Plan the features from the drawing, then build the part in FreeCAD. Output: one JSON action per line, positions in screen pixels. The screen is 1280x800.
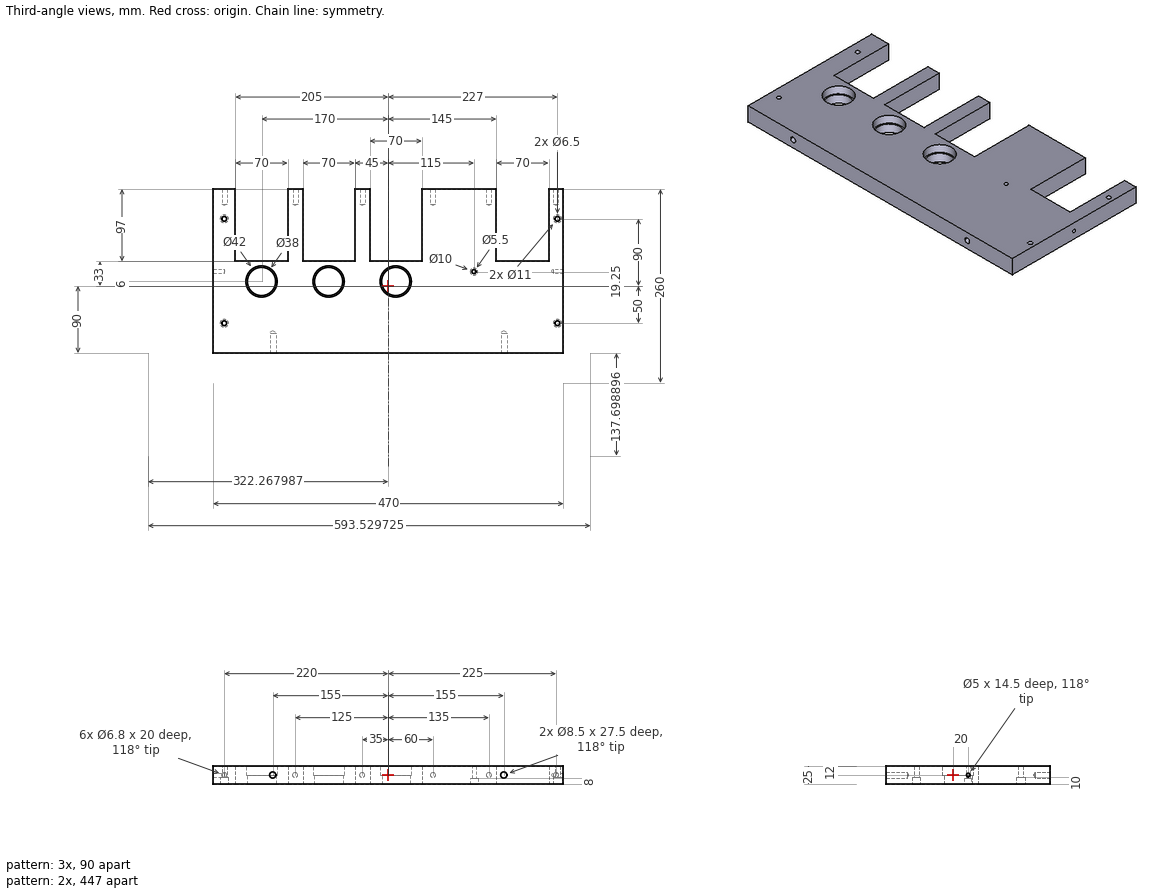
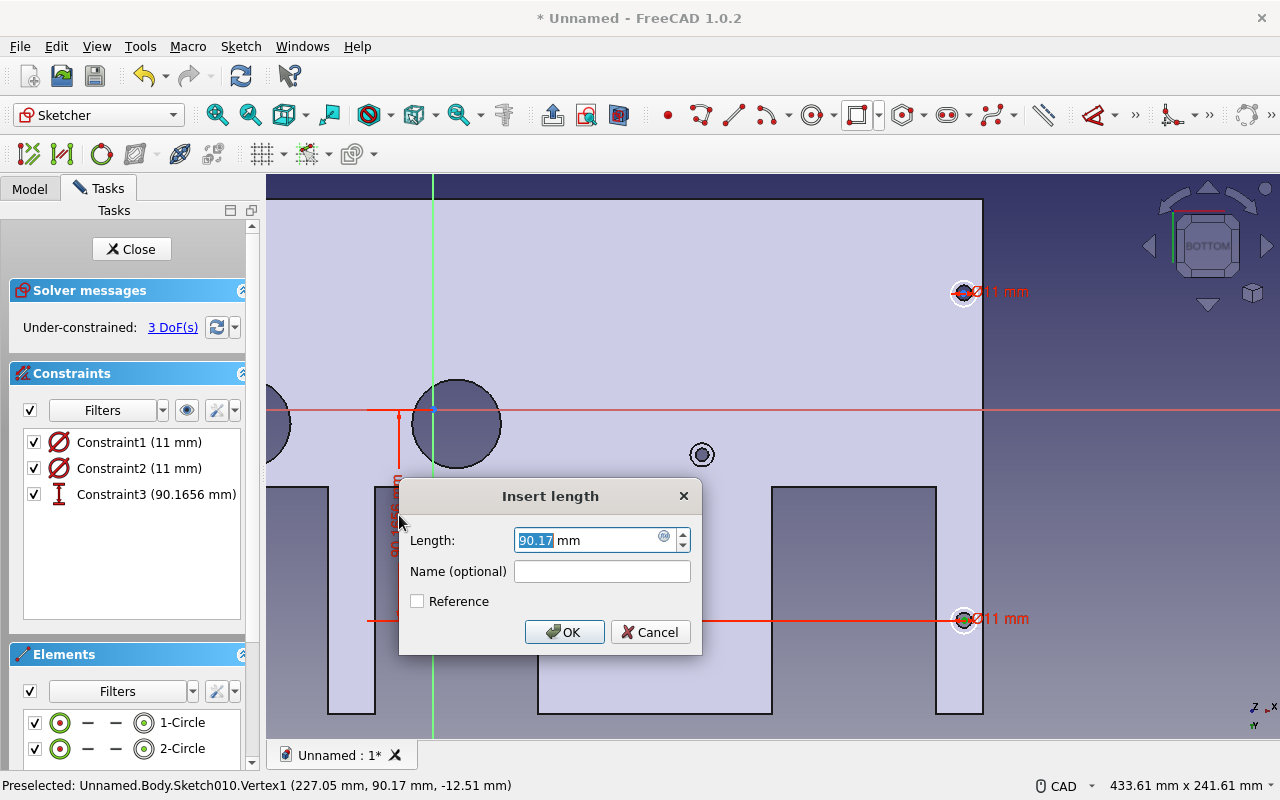
{"action": "type", "text": "90"}
{"action": "key", "text": "Return"}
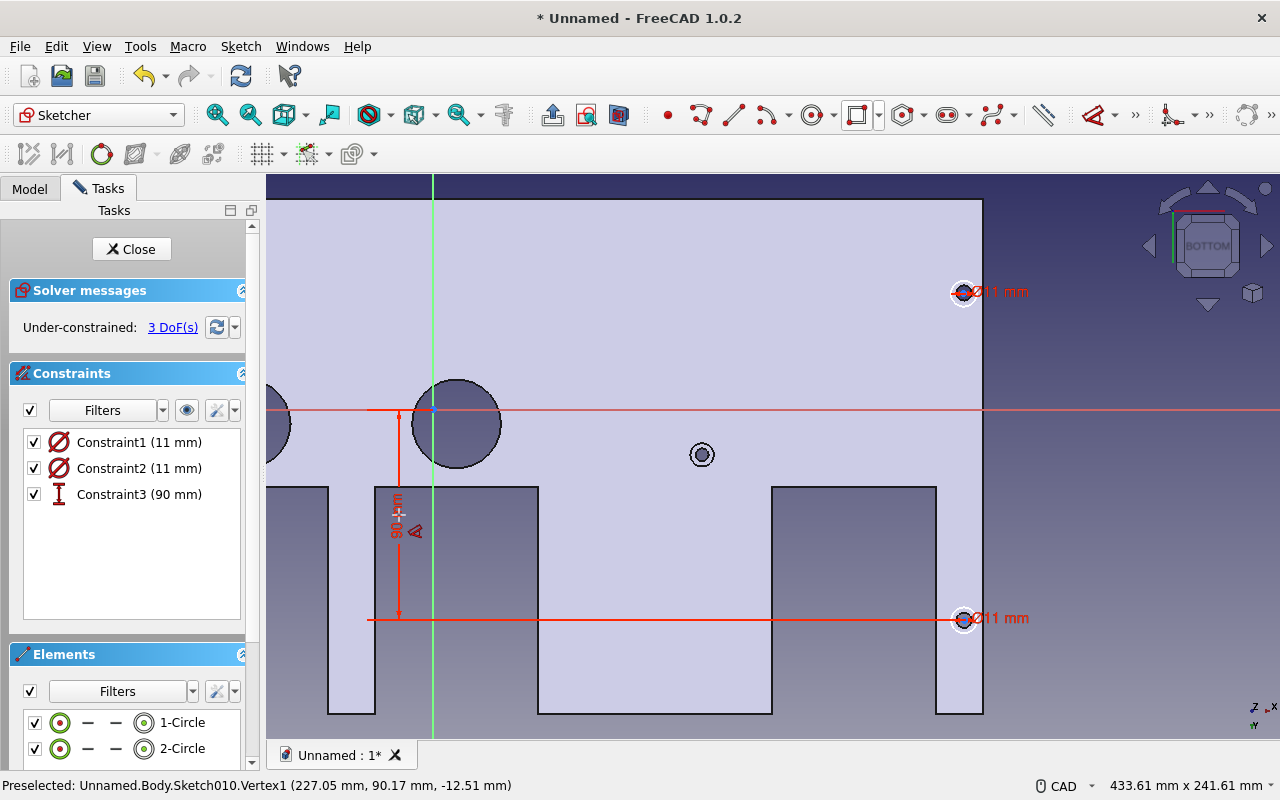
{"action": "left_click", "coordinate": [964, 294]}
{"action": "left_click", "coordinate": [399, 352]}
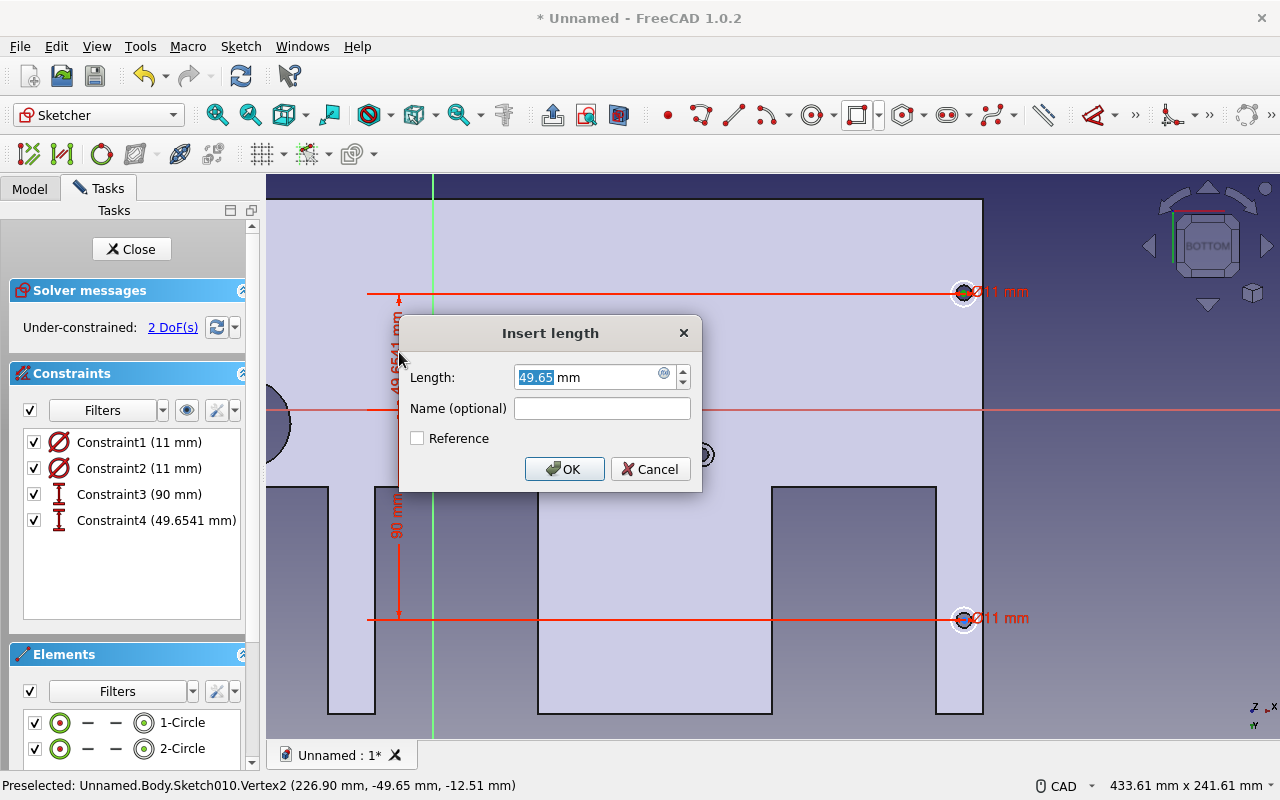
{"action": "type", "text": "50"}
{"action": "key", "text": "Return"}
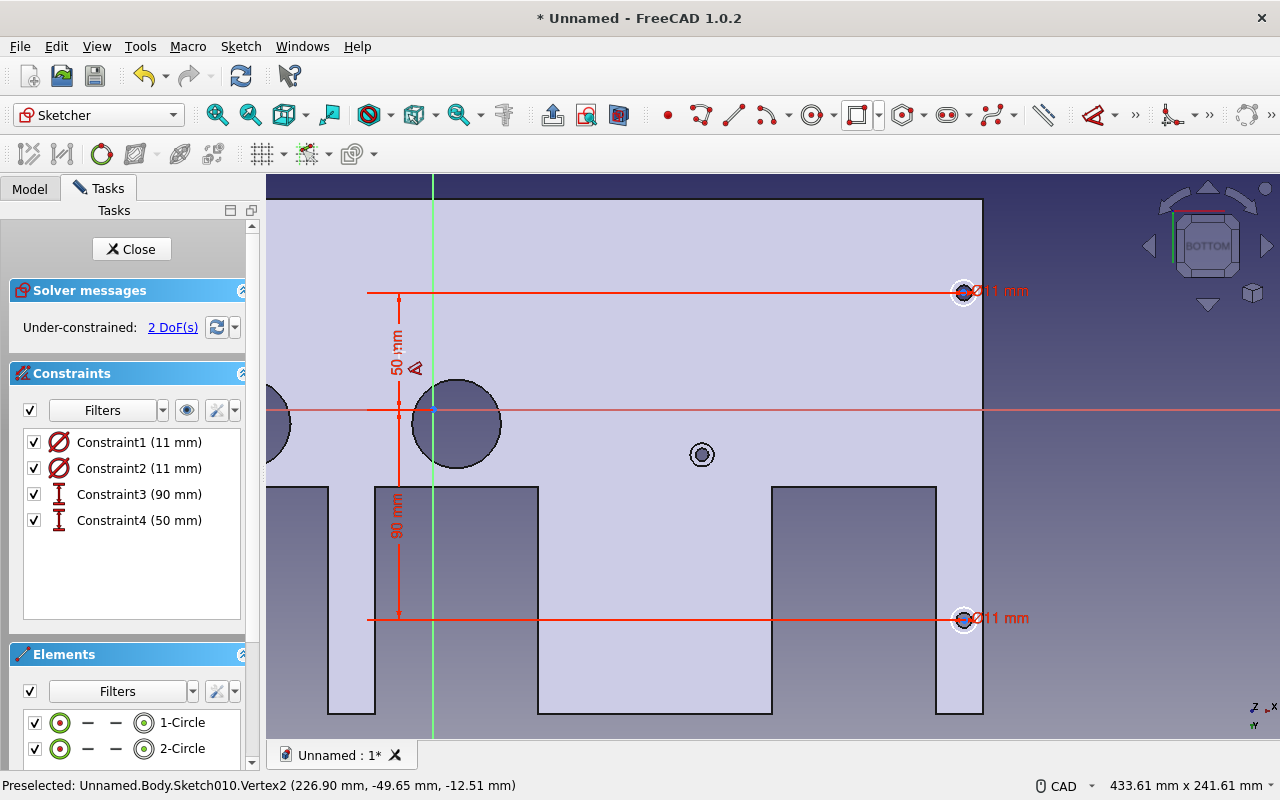
{"action": "left_click", "coordinate": [964, 620]}
{"action": "left_click", "coordinate": [699, 654]}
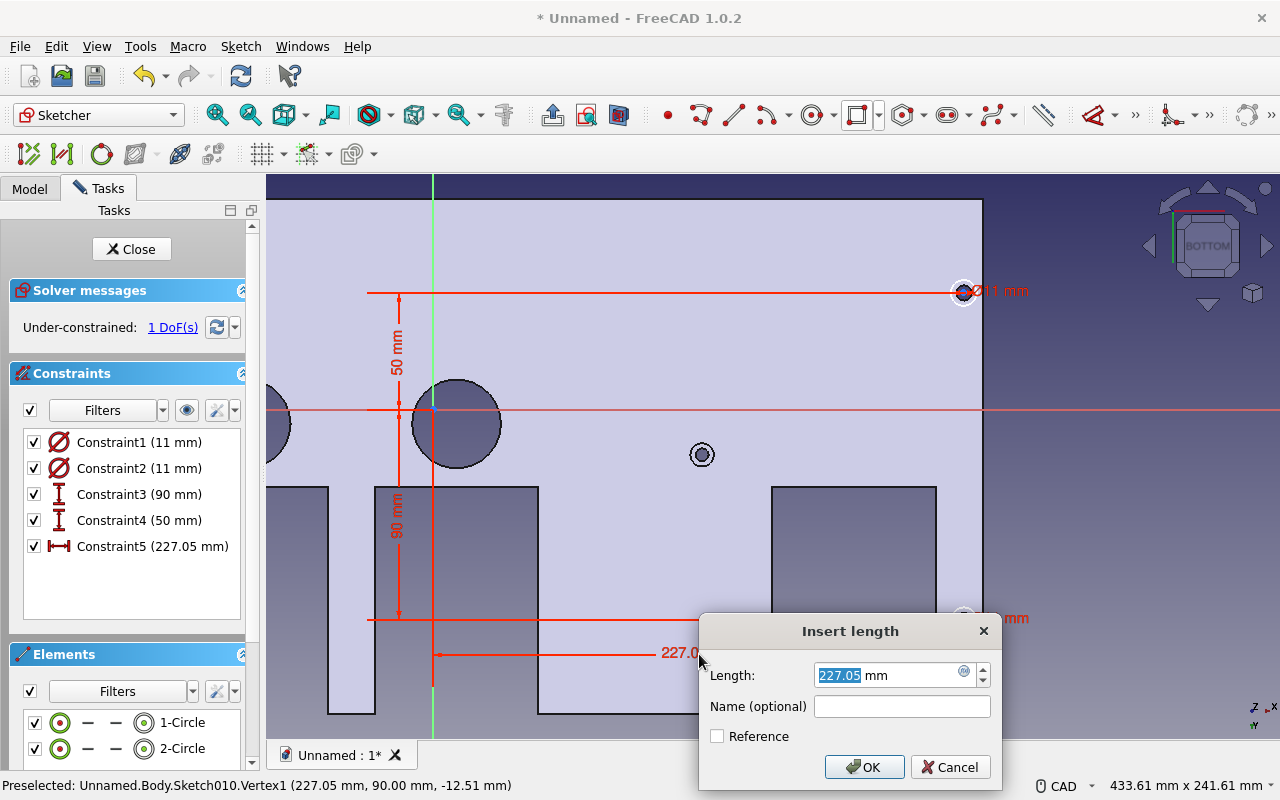
{"action": "type", "text": "227"}
{"action": "key", "text": "Return"}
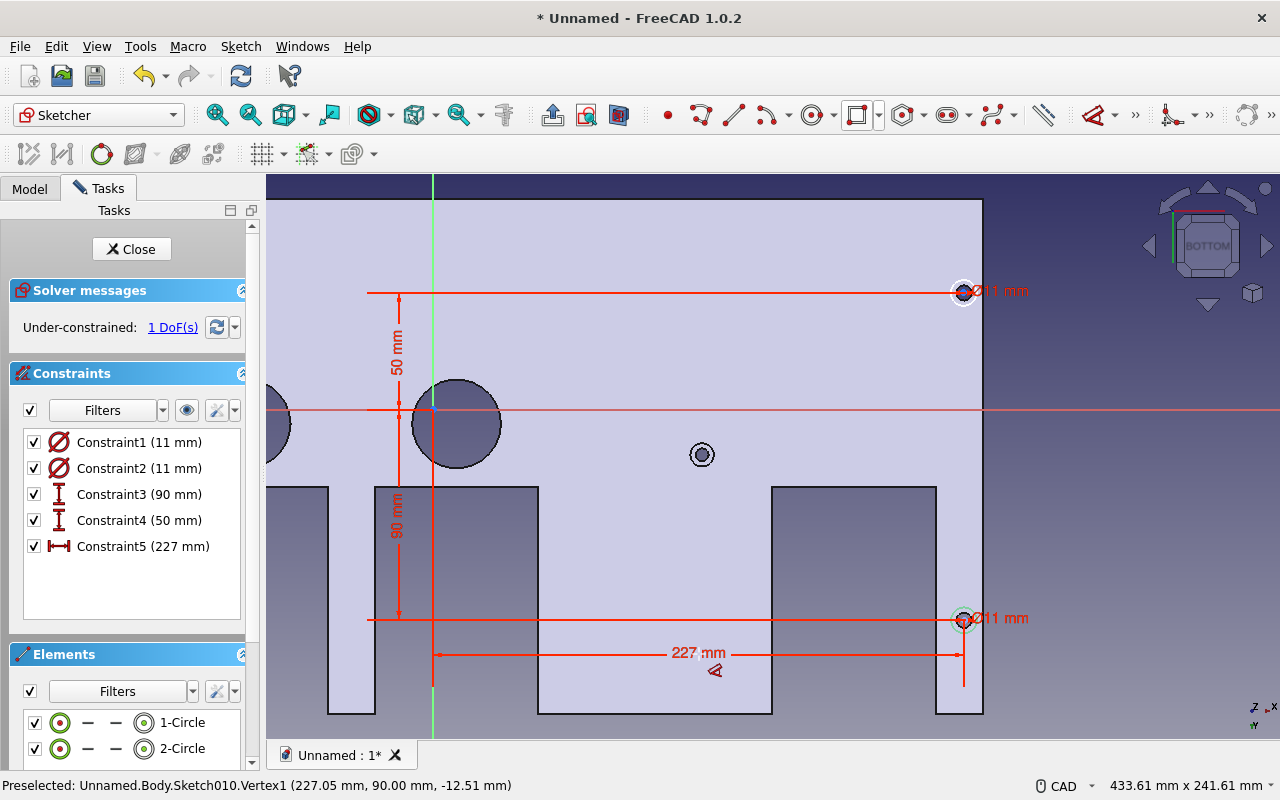
{"action": "left_click", "coordinate": [964, 293]}
{"action": "left_click", "coordinate": [698, 259]}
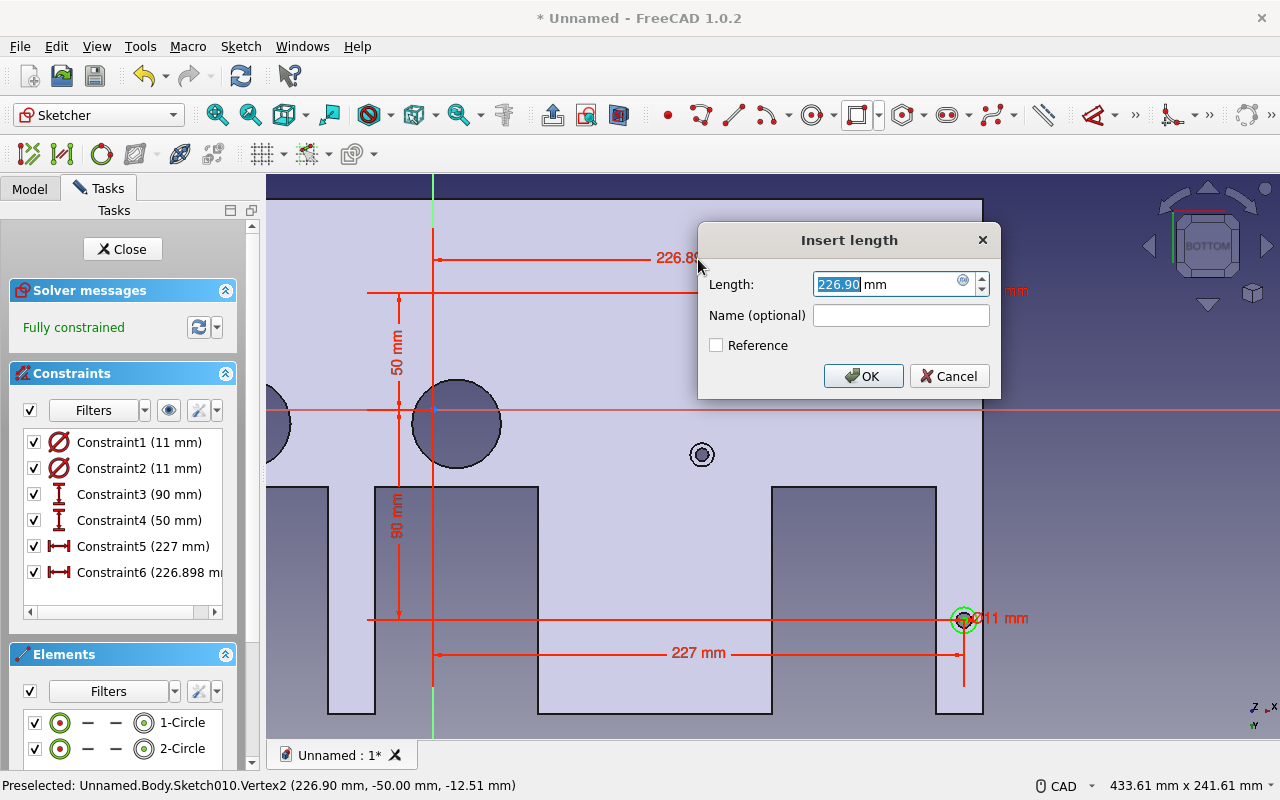
{"action": "type", "text": "227"}
{"action": "key", "text": "Return"}
{"action": "key", "text": "Escape"}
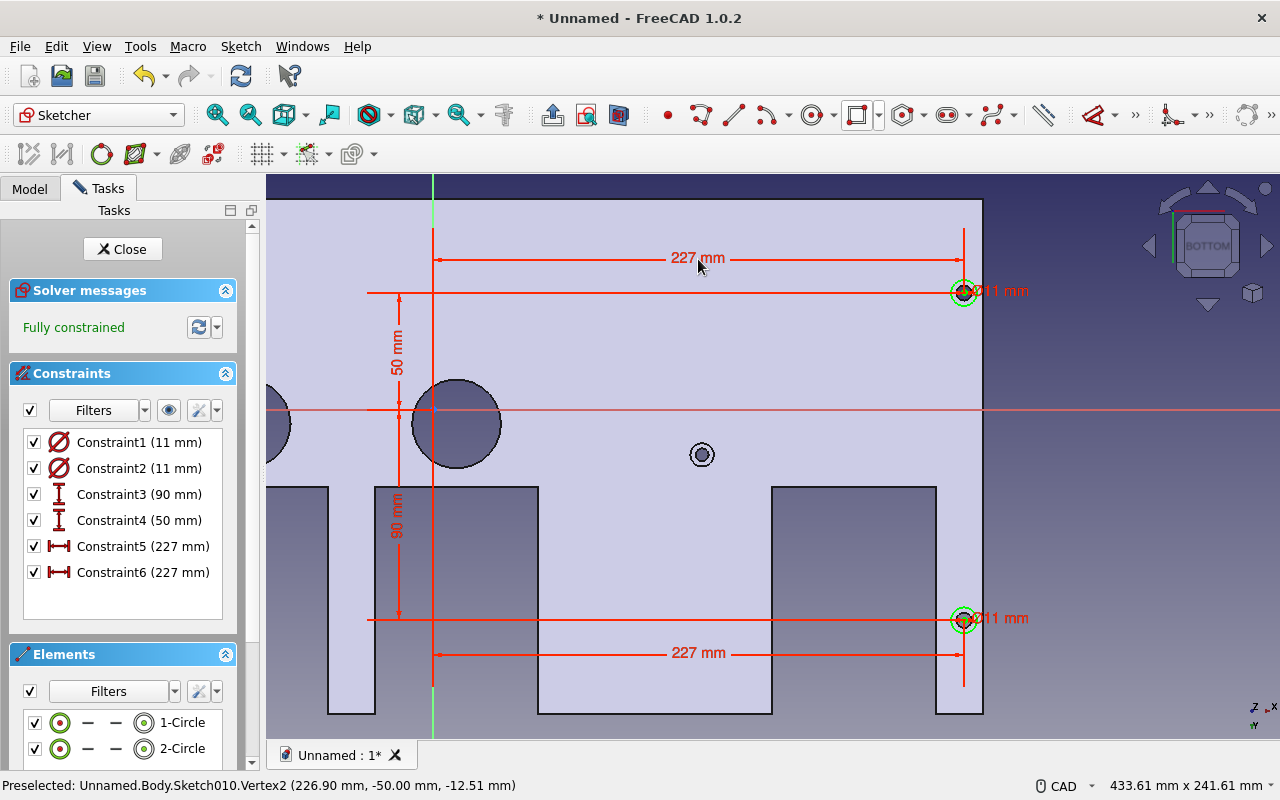
{"action": "left_click", "coordinate": [123, 249]}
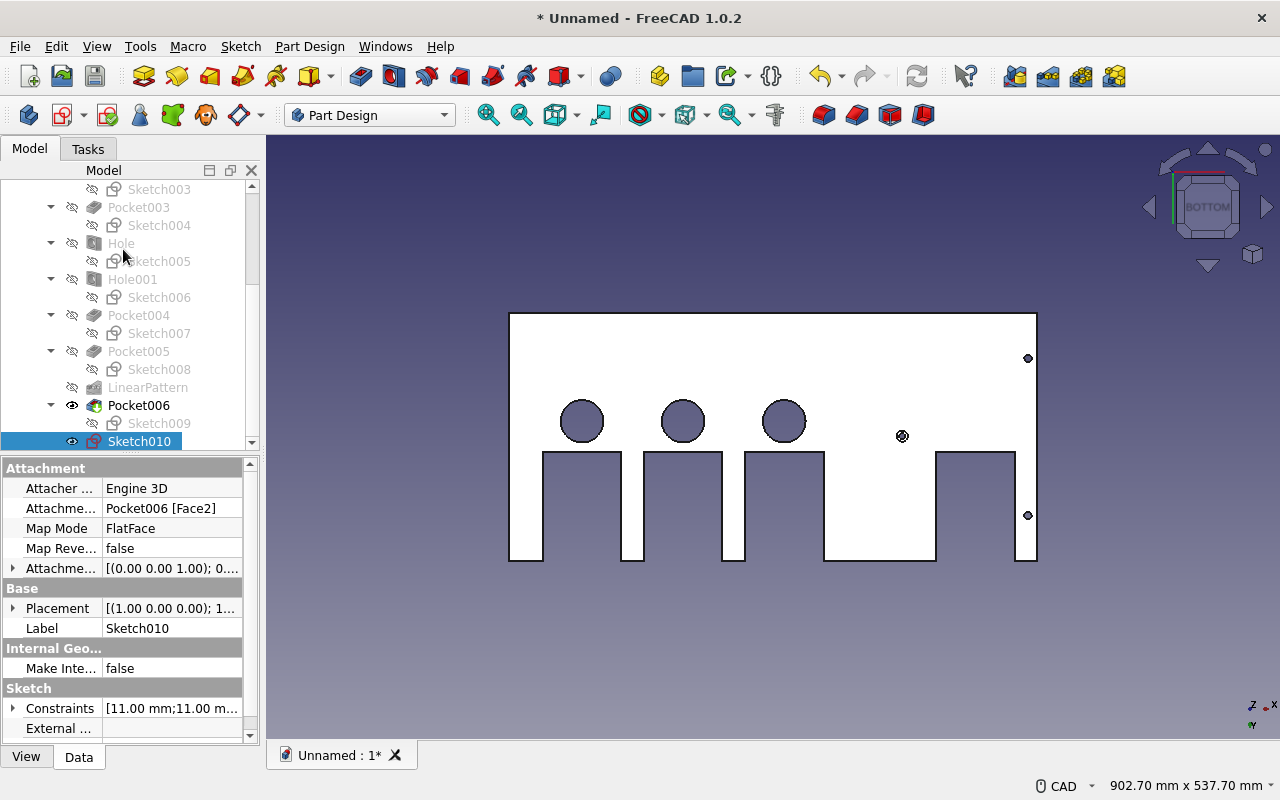
{"action": "left_click", "coordinate": [361, 76]}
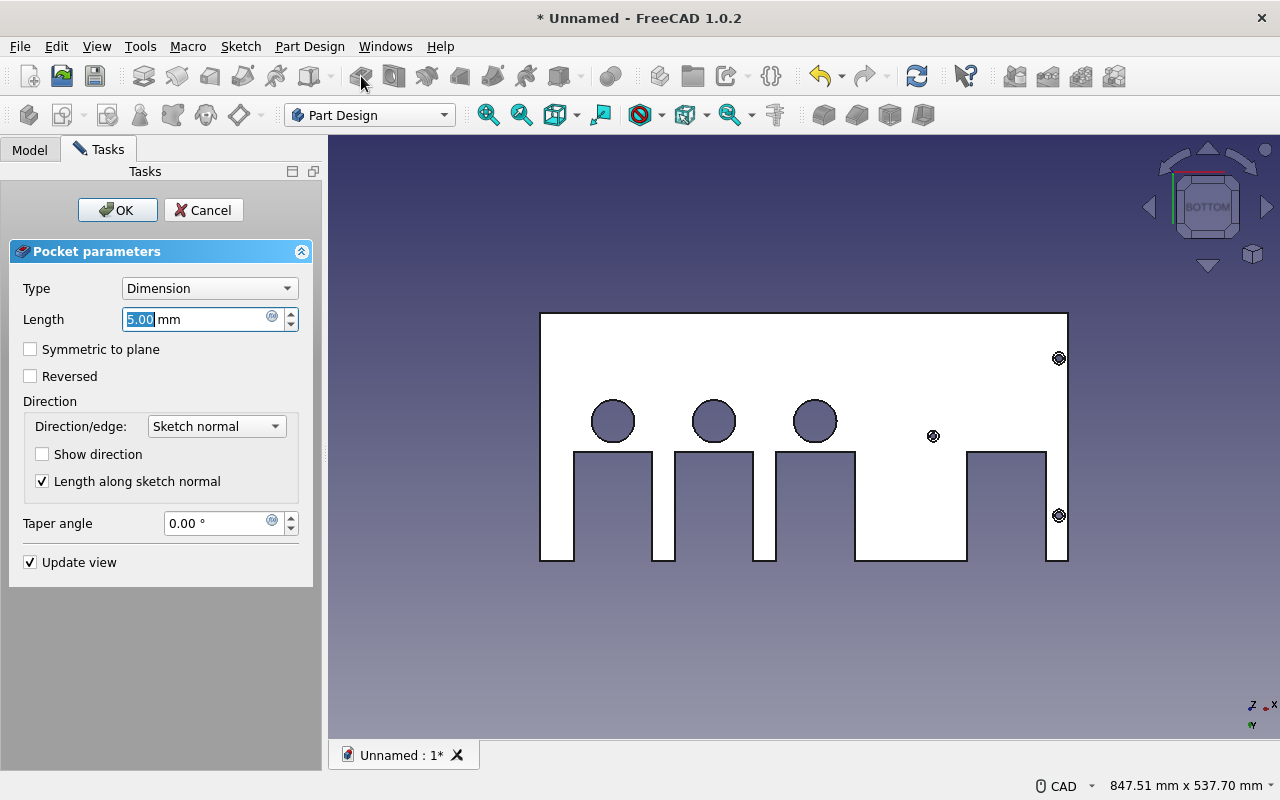
{"action": "type", "text": "10"}
{"action": "key", "text": "Tab"}